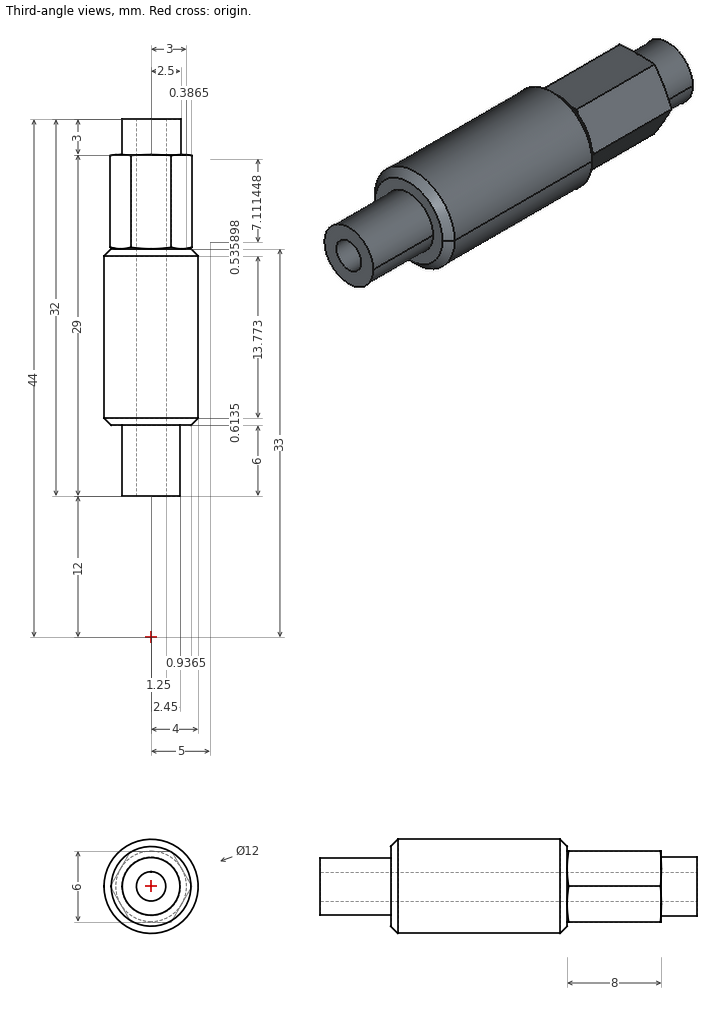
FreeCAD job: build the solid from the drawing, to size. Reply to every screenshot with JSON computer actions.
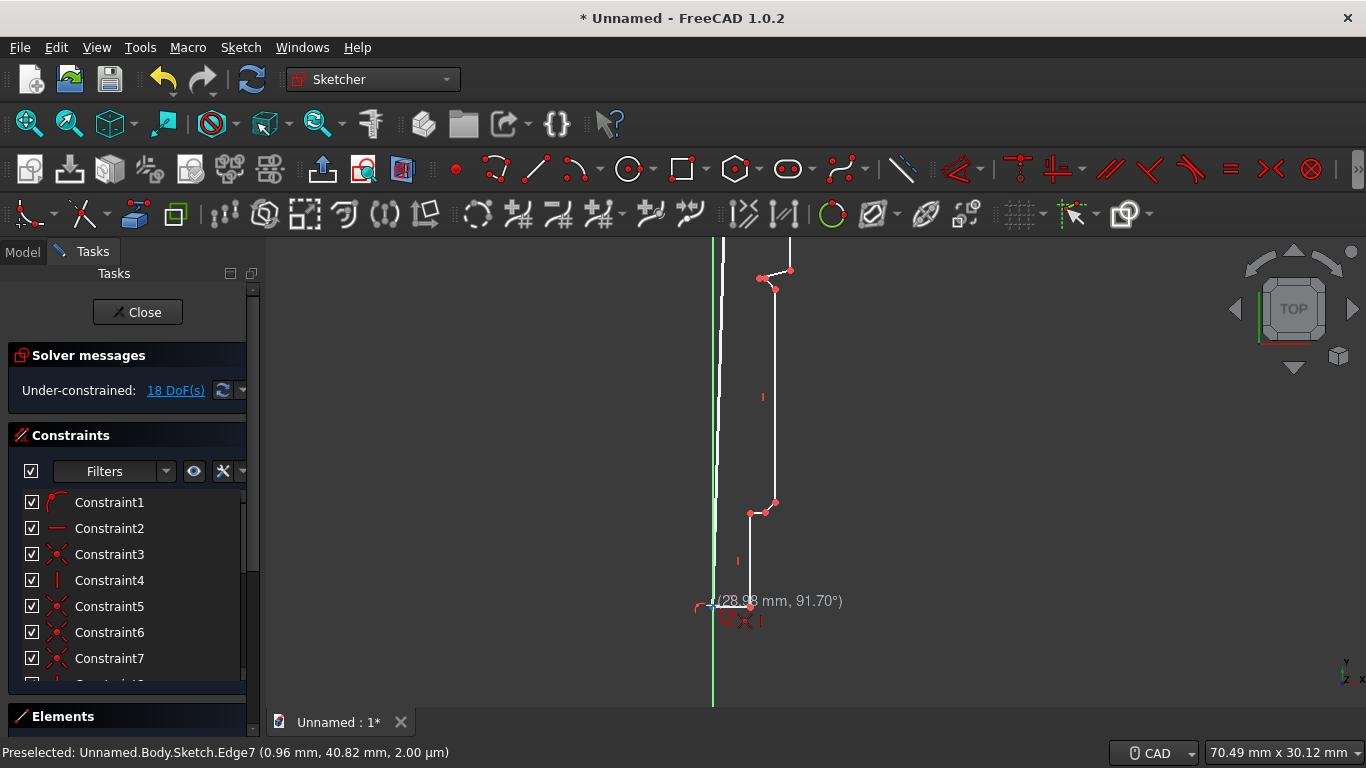
{"action": "left_click", "coordinate": [713, 607]}
{"action": "key", "text": "Escape"}
{"action": "key", "text": "Escape"}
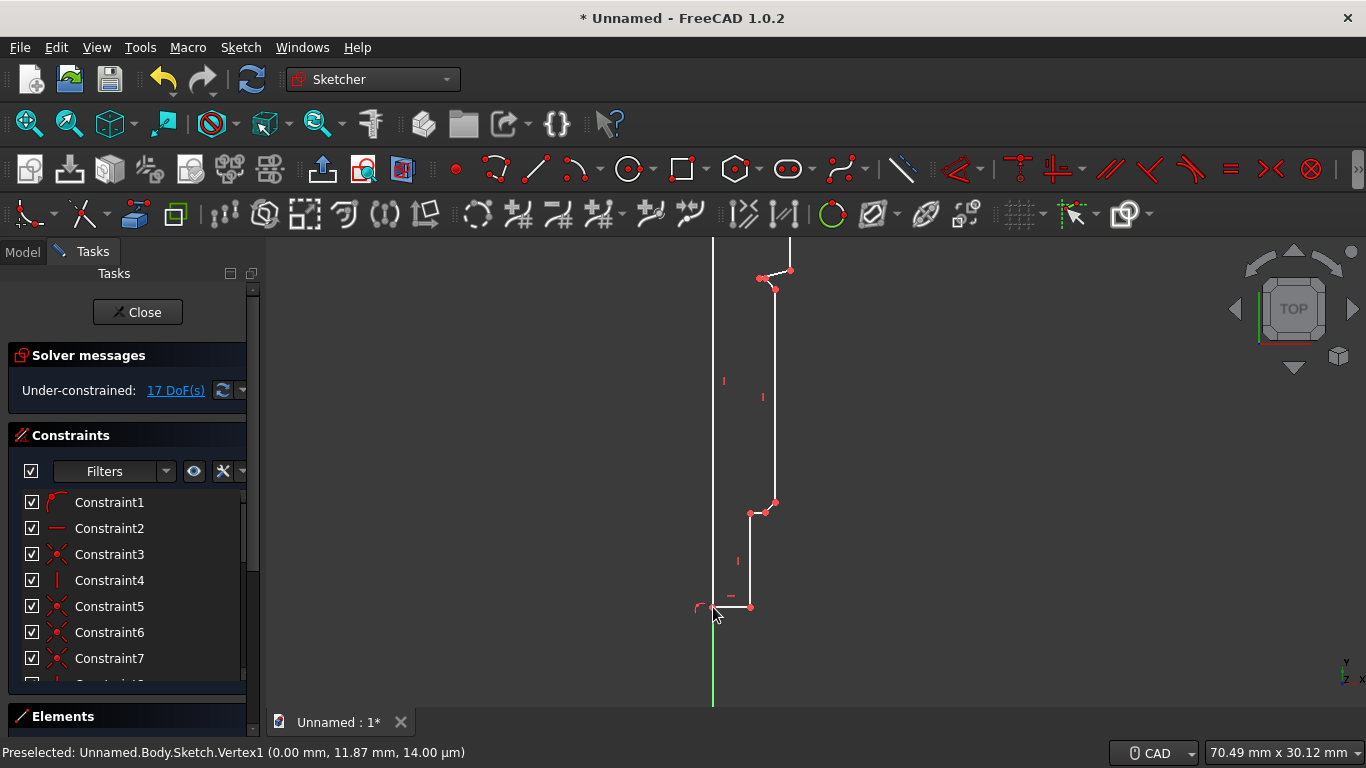
{"action": "scroll", "coordinate": [758, 513], "scroll_direction": "up", "scroll_amount": 3}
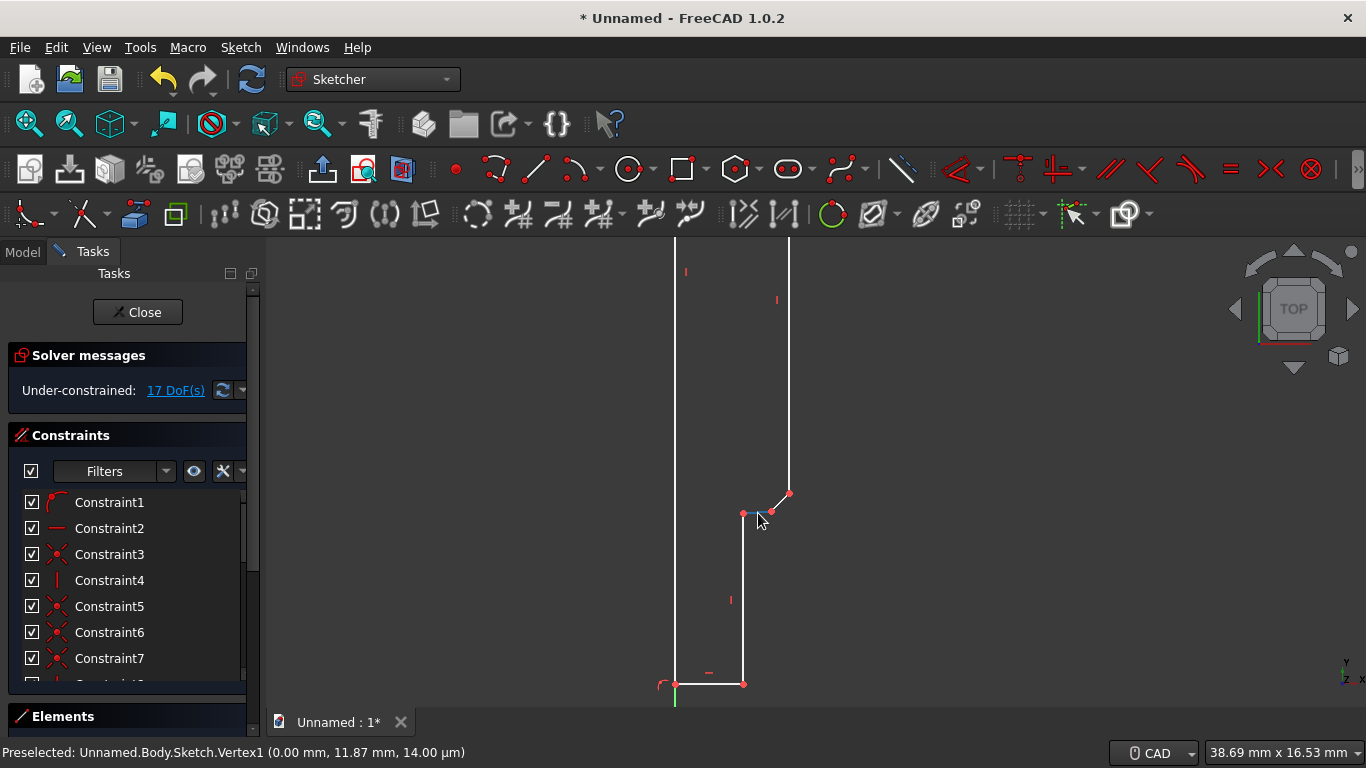
{"action": "left_click", "coordinate": [757, 513]}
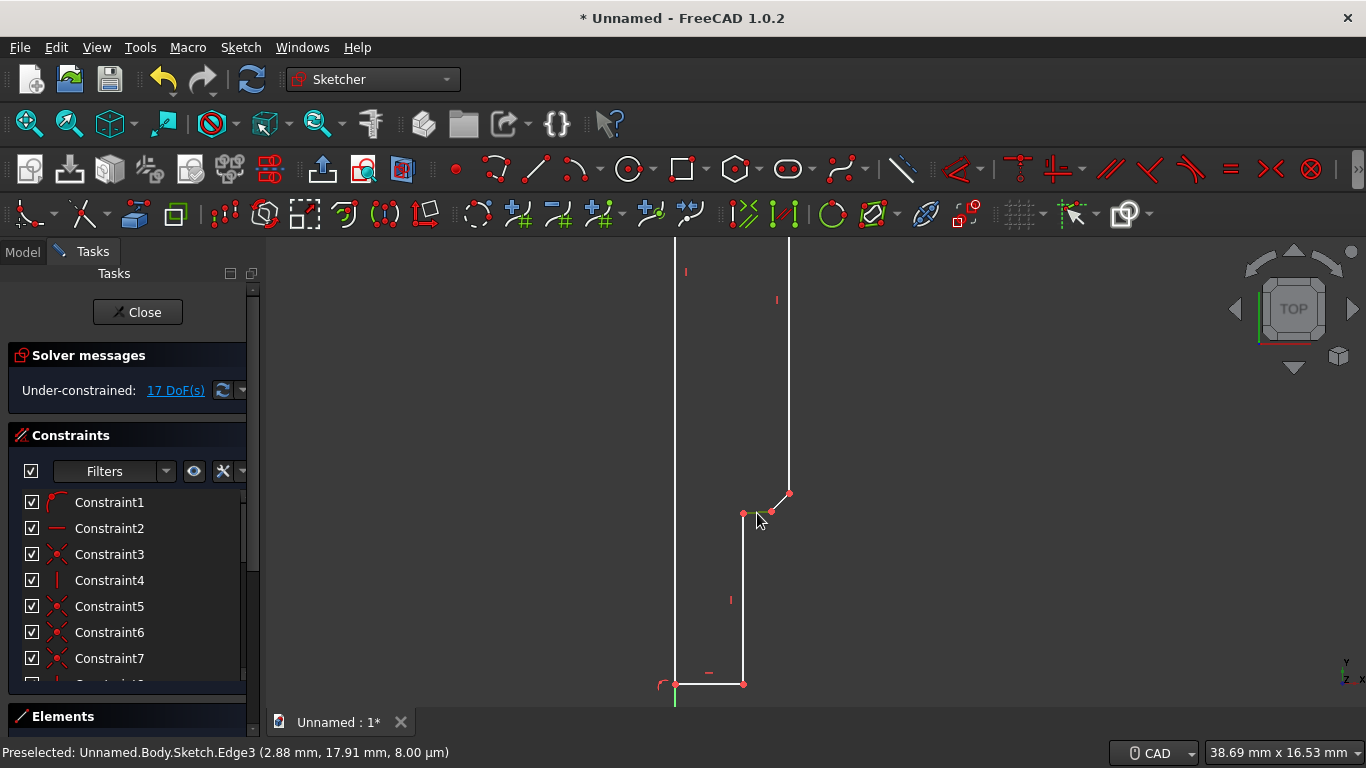
{"action": "left_click", "coordinate": [1084, 170]}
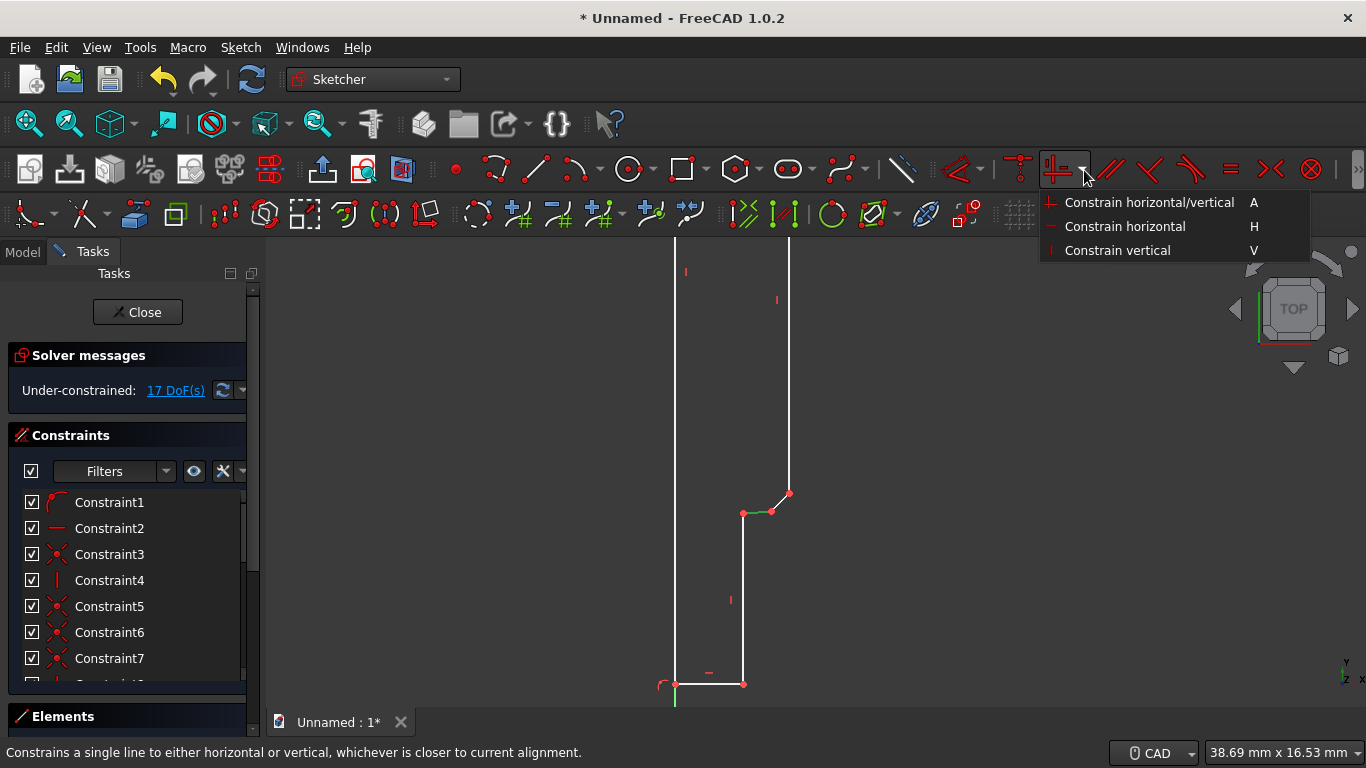
{"action": "left_click", "coordinate": [1175, 226]}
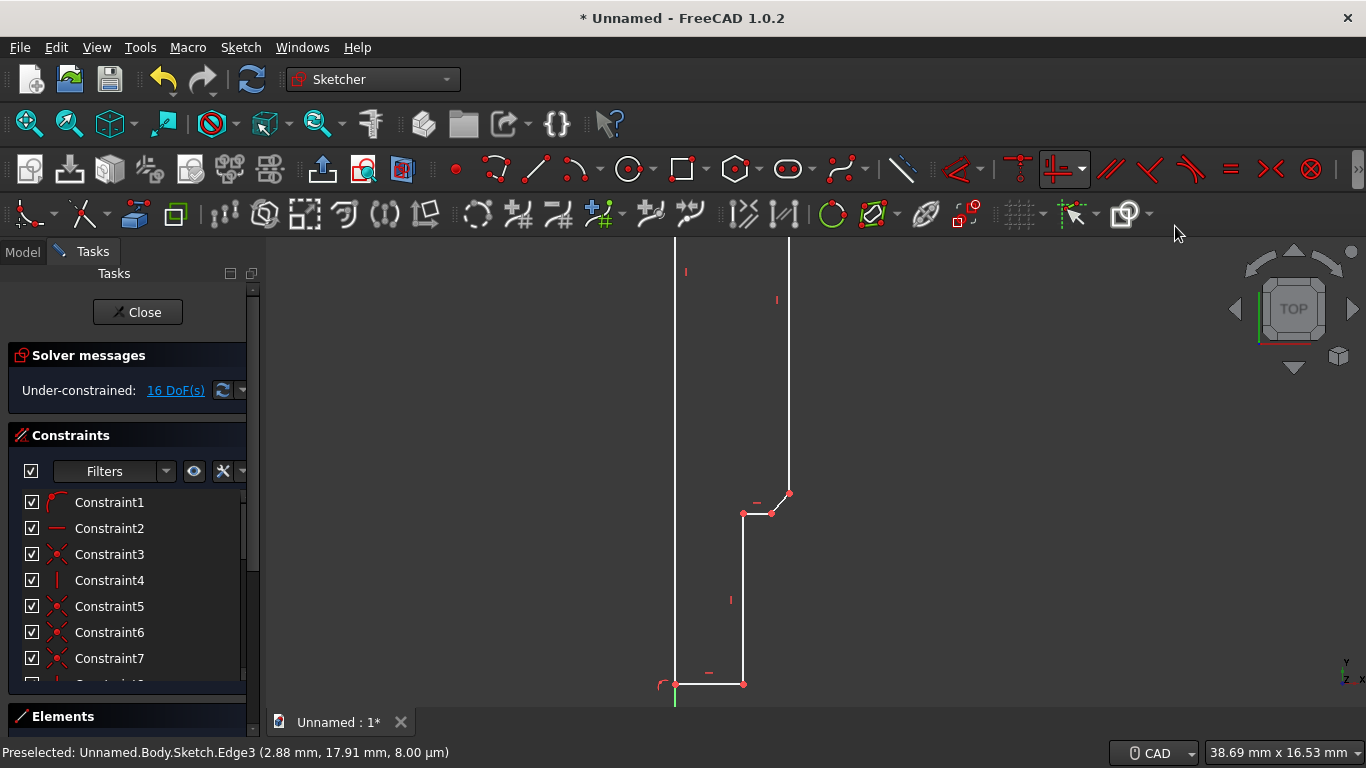
{"action": "scroll", "coordinate": [748, 483], "scroll_direction": "down", "scroll_amount": 7}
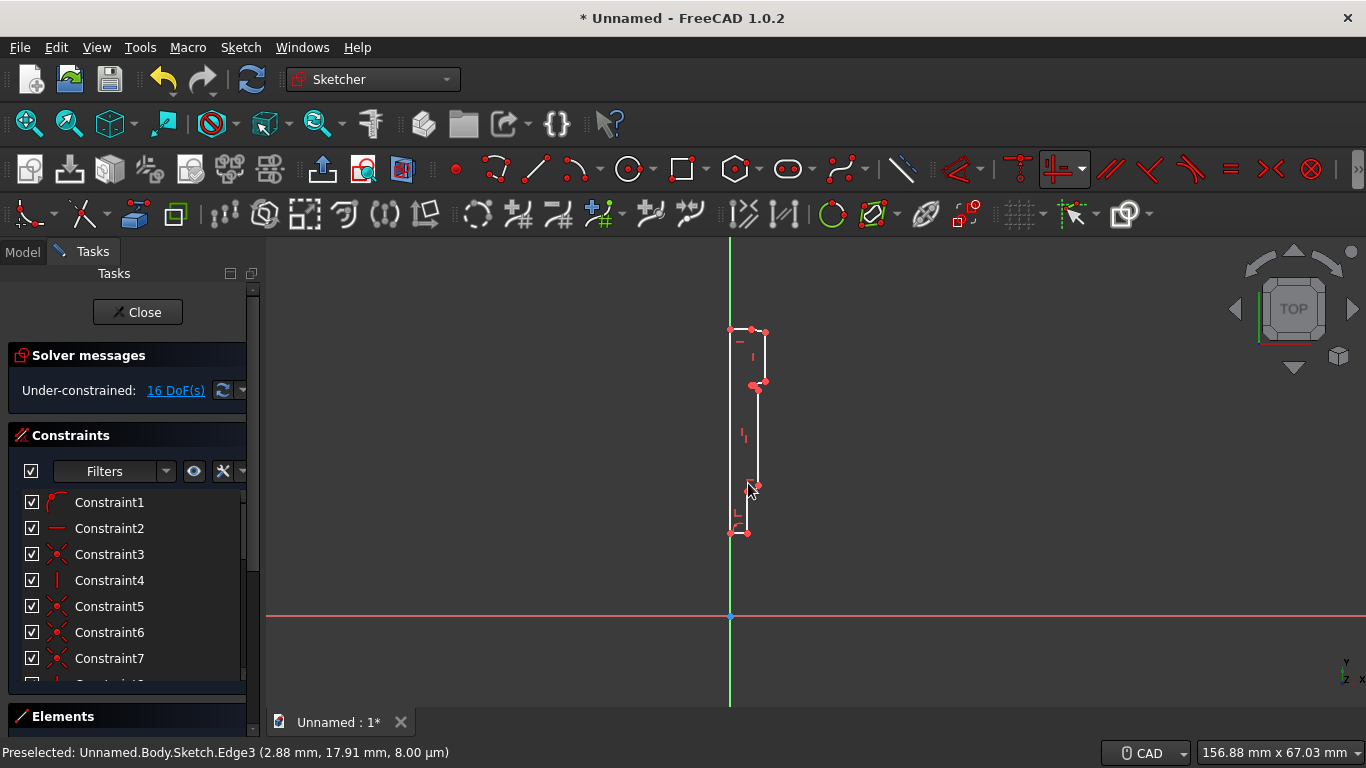
{"action": "scroll", "coordinate": [753, 385], "scroll_direction": "up", "scroll_amount": 14}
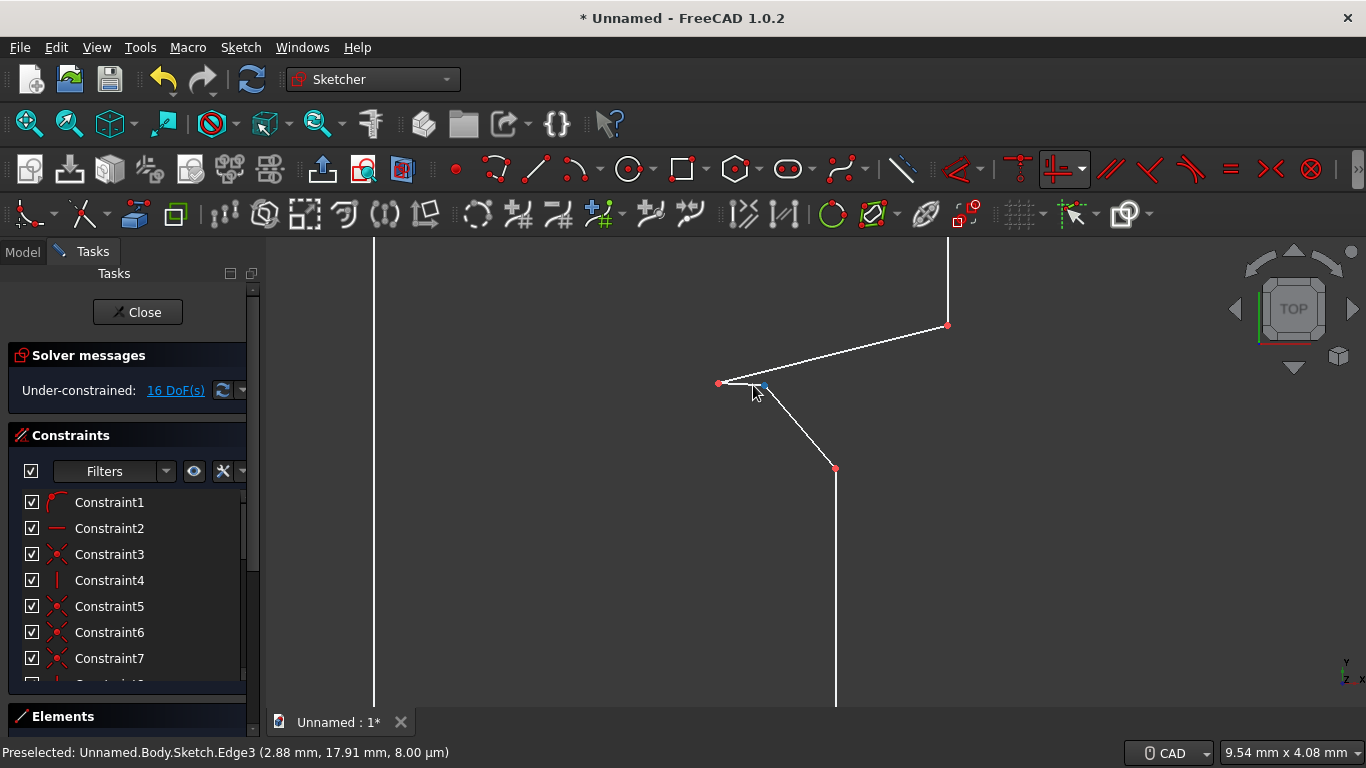
{"action": "left_click", "coordinate": [751, 385]}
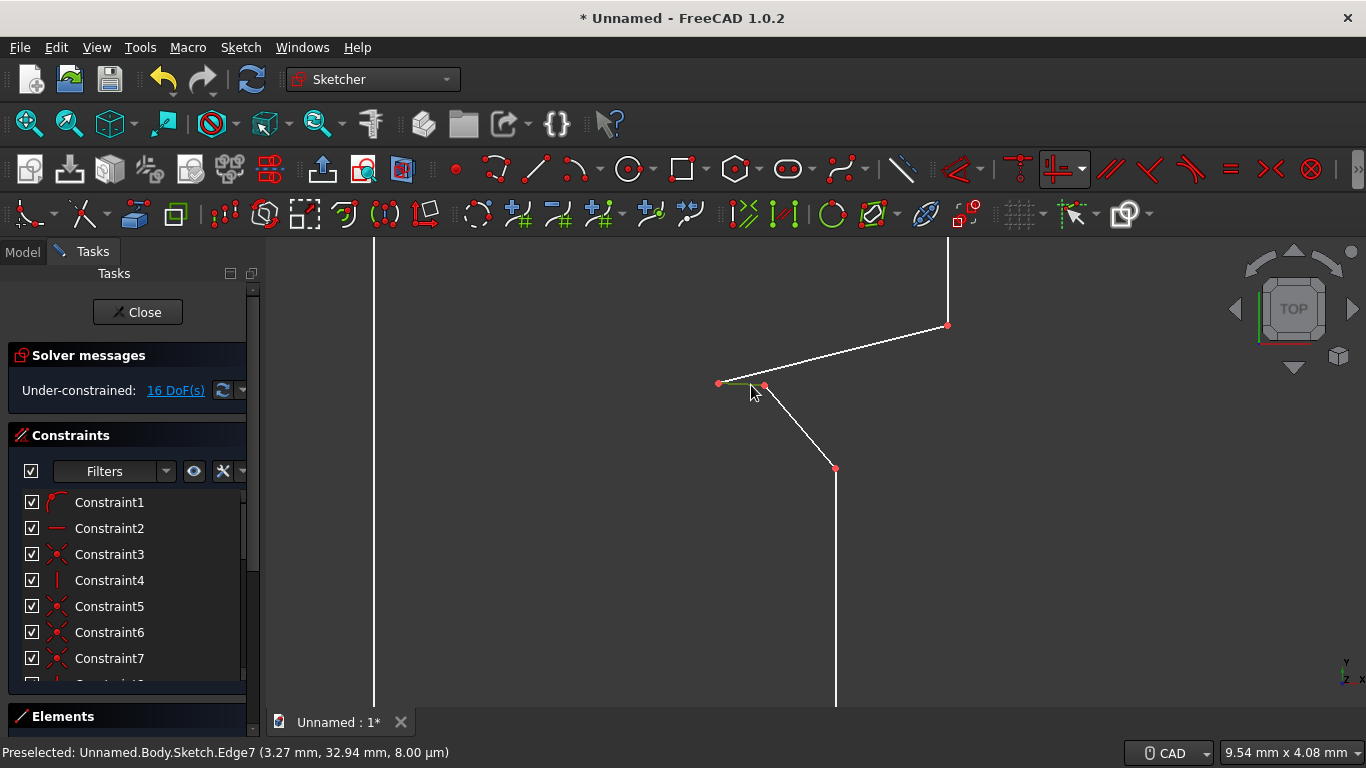
{"action": "key", "text": "h"}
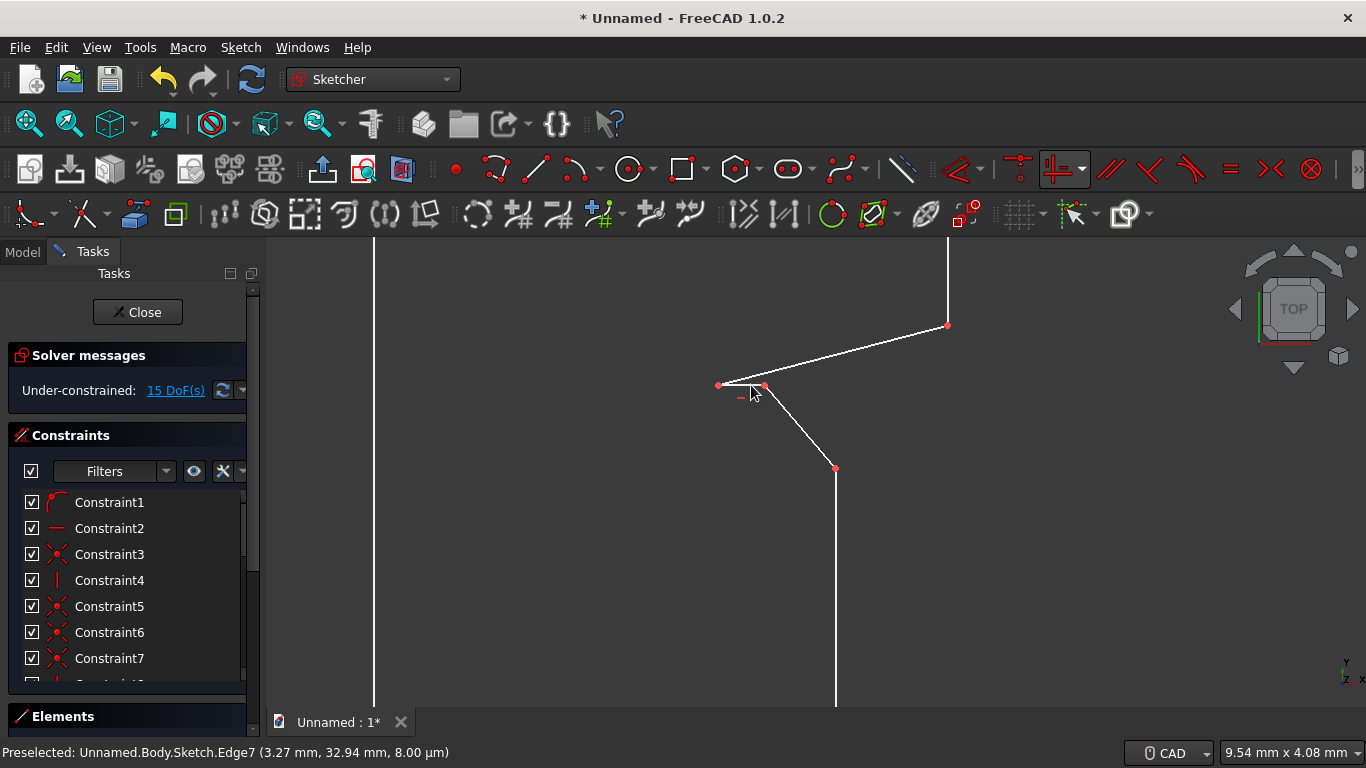
{"action": "left_click", "coordinate": [956, 170]}